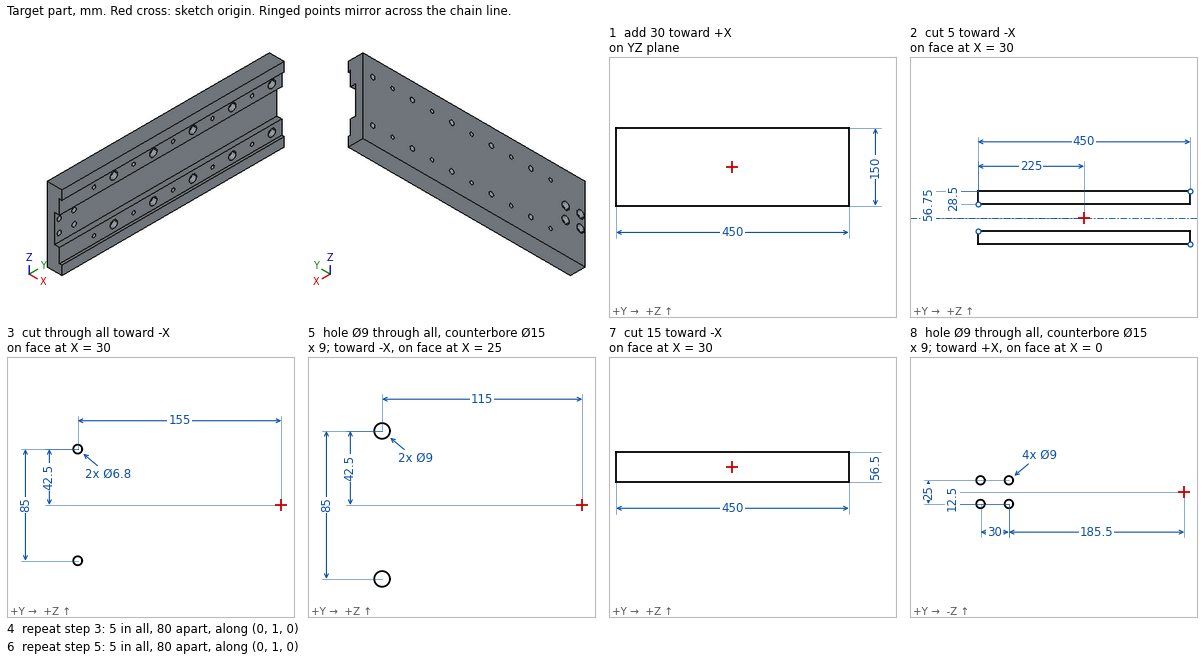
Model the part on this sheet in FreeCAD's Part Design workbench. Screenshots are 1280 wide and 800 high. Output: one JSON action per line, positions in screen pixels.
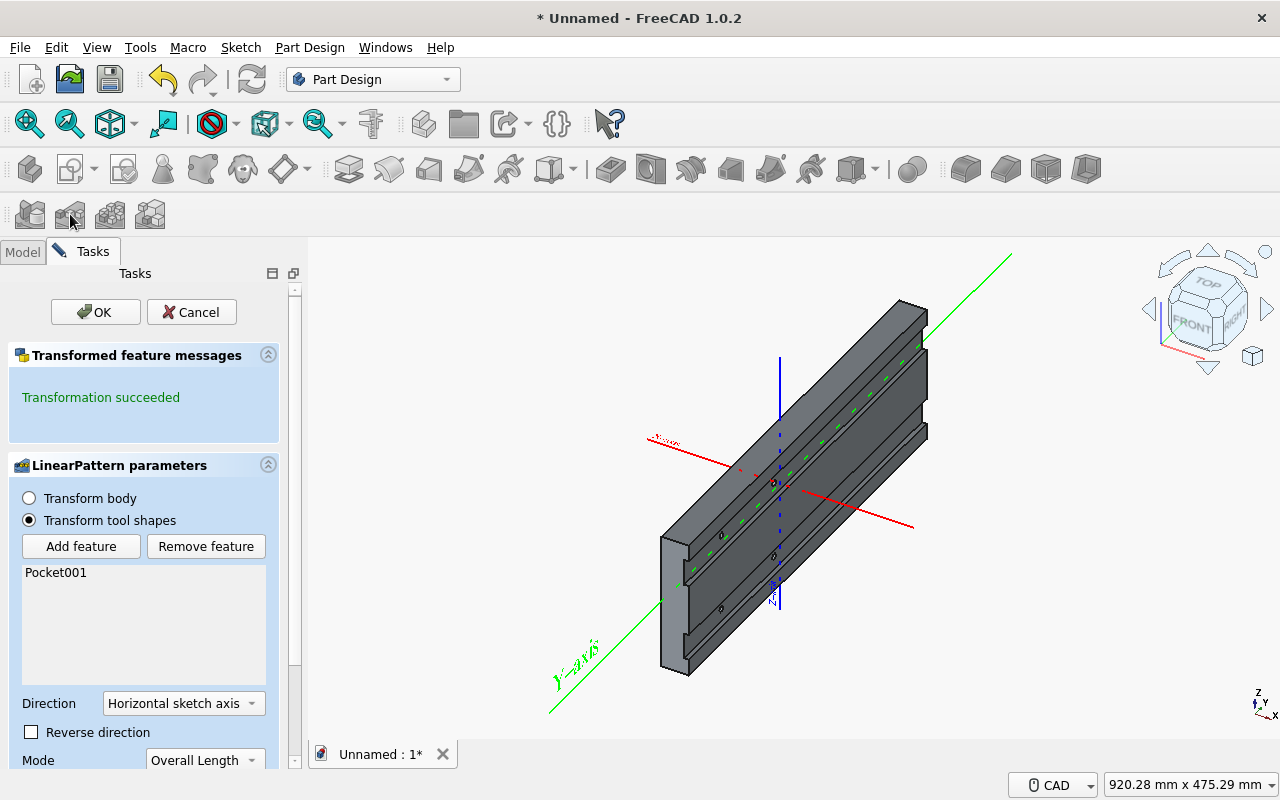
{"action": "left_click", "coordinate": [184, 704]}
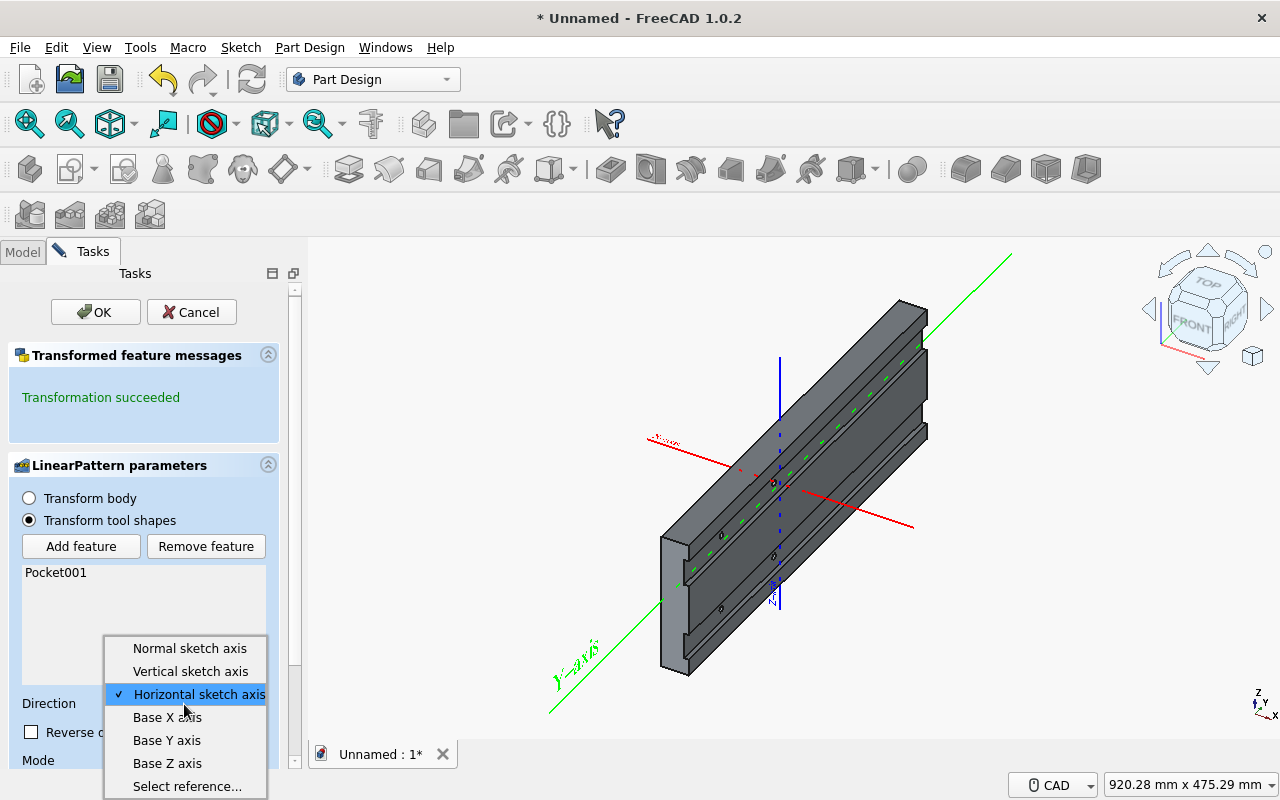
{"action": "left_click", "coordinate": [184, 740]}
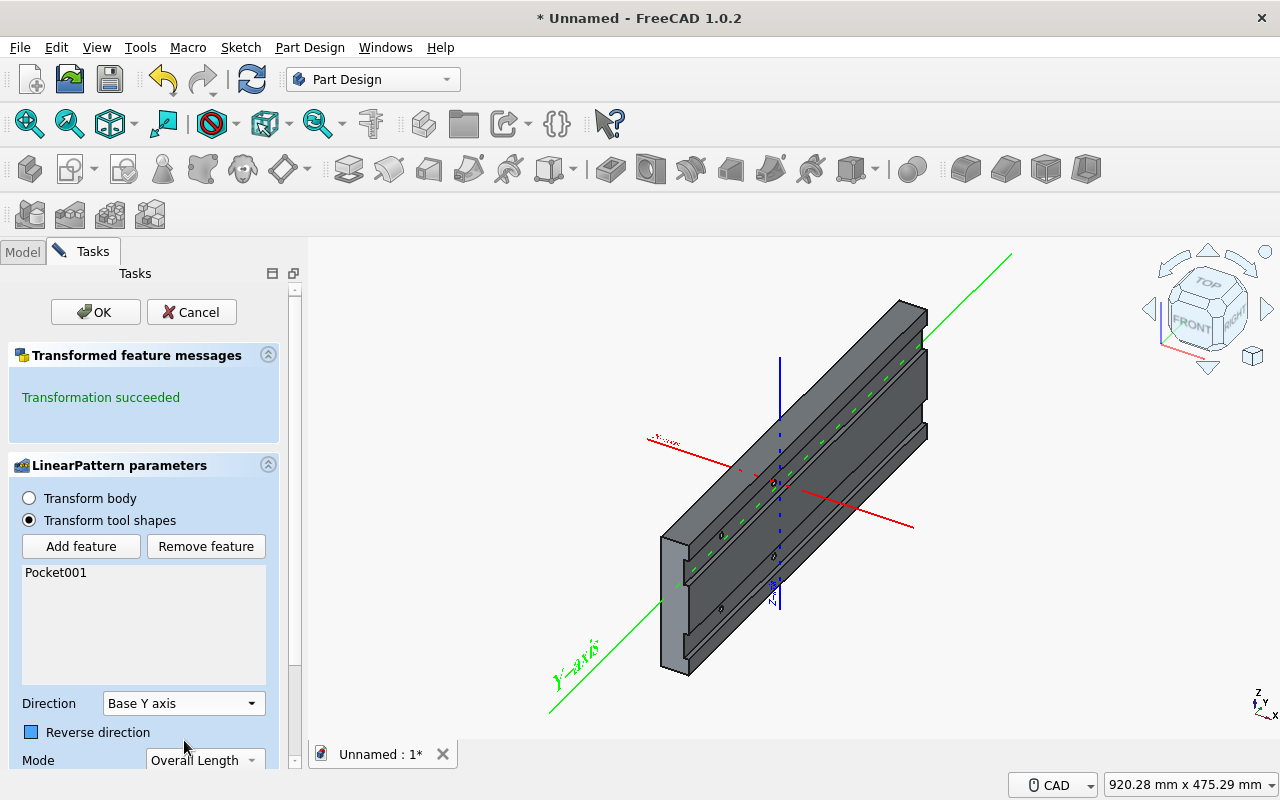
{"action": "scroll", "coordinate": [295, 526], "scroll_direction": "down", "scroll_amount": 2}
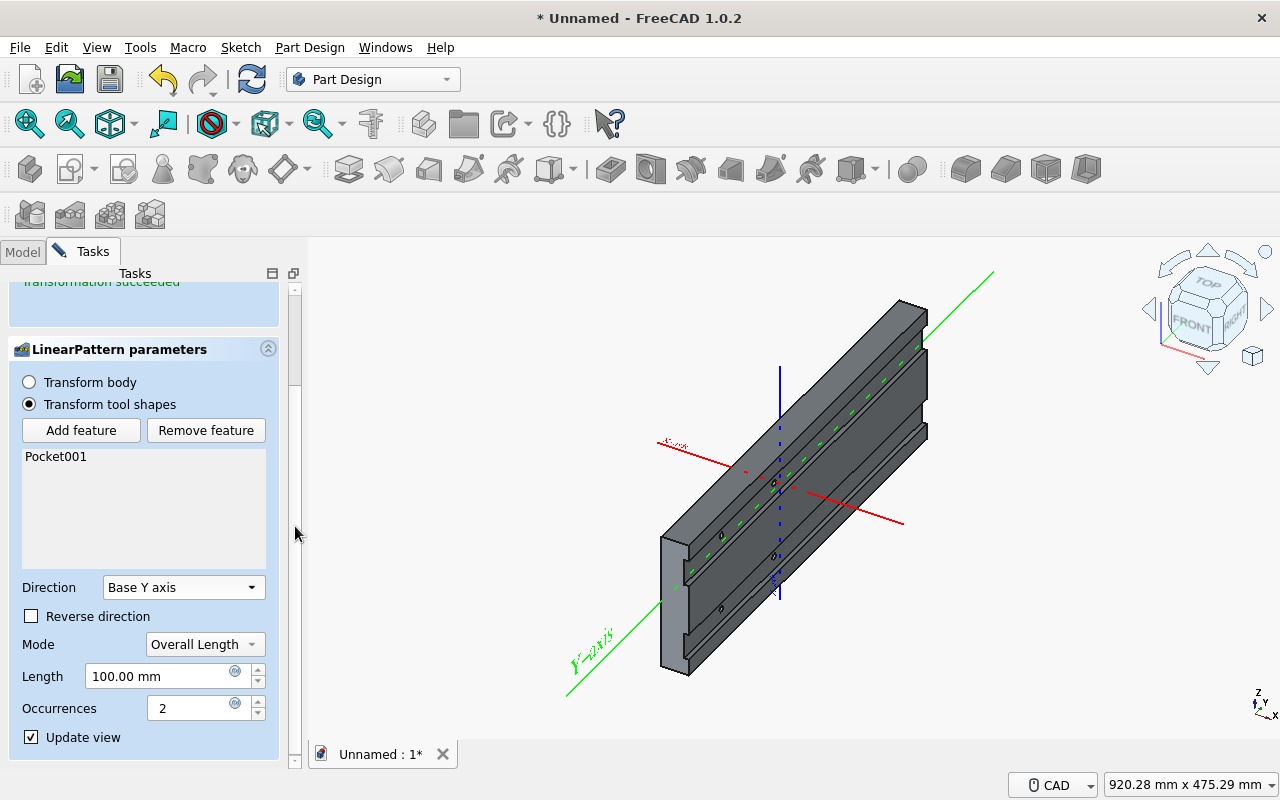
{"action": "left_click", "coordinate": [206, 644]}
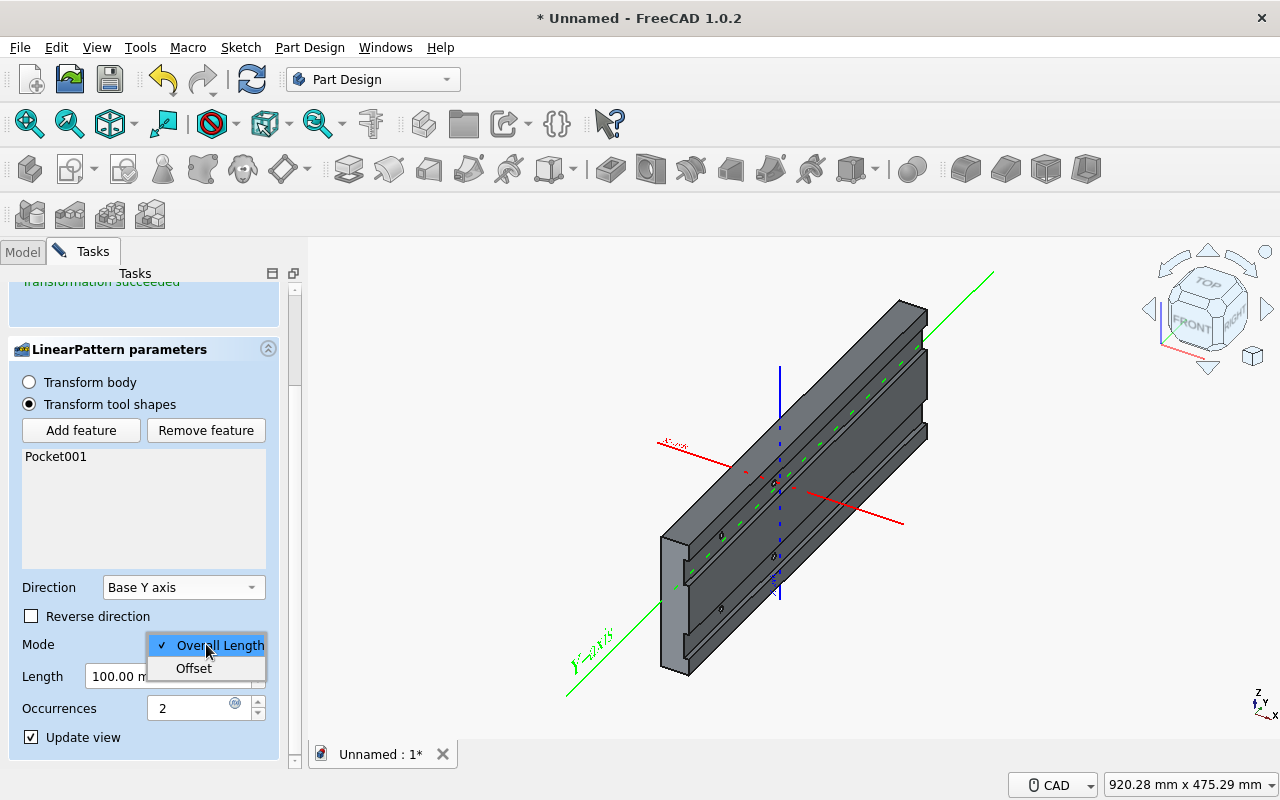
{"action": "left_click", "coordinate": [206, 668]}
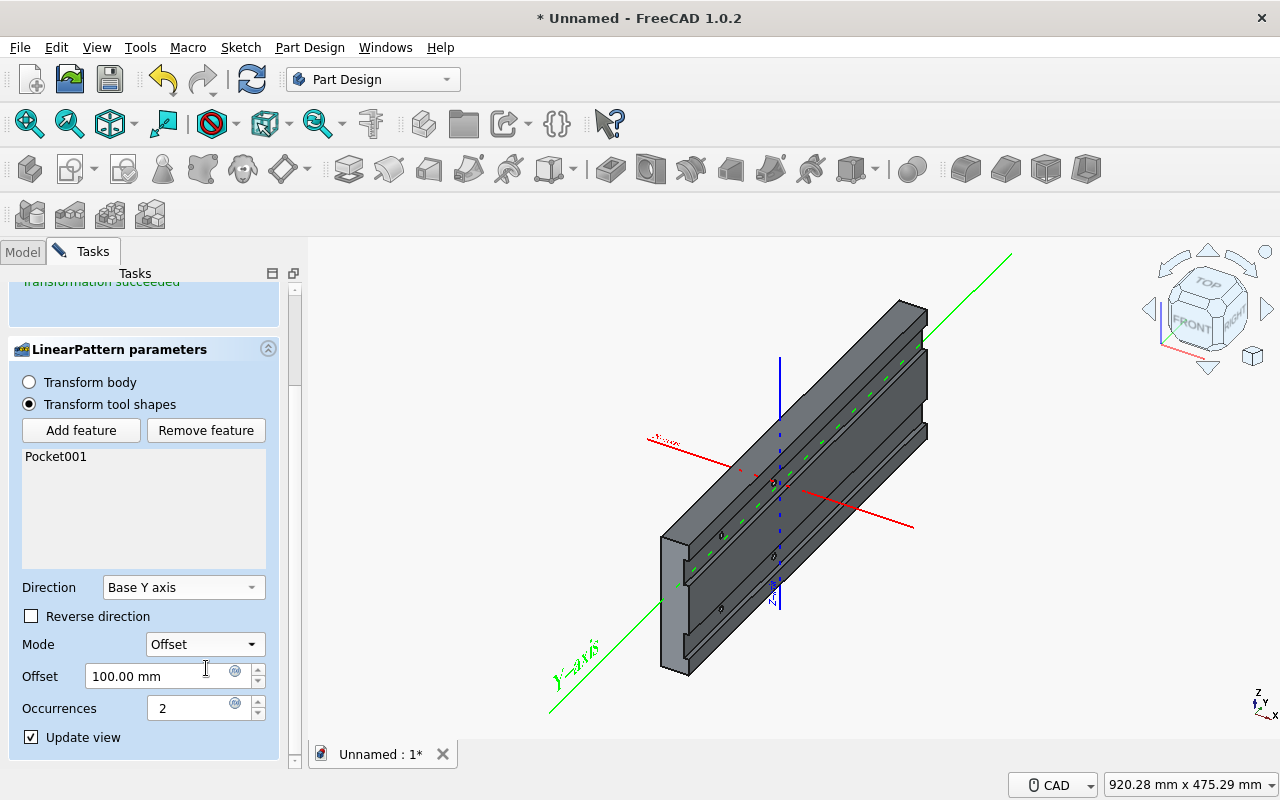
{"action": "triple_click", "coordinate": [168, 676]}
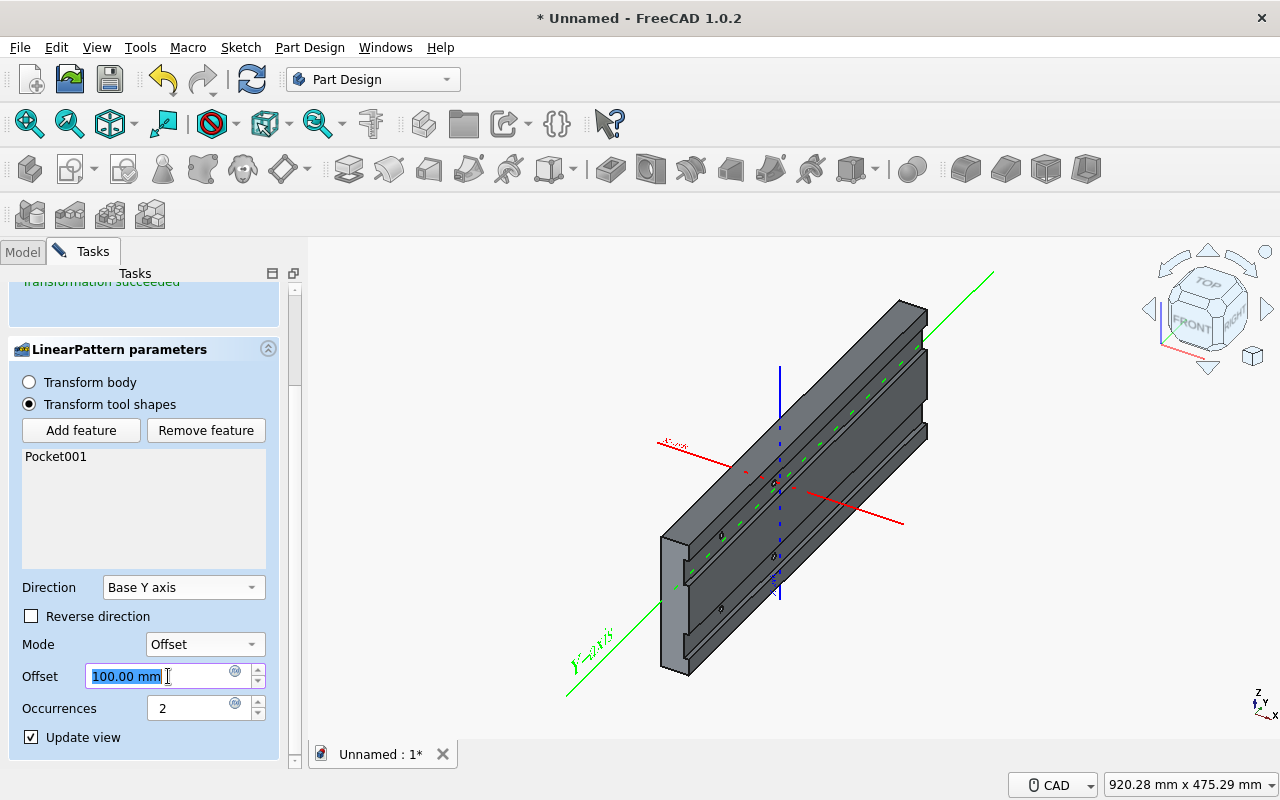
{"action": "type", "text": "80"}
{"action": "key", "text": "Tab"}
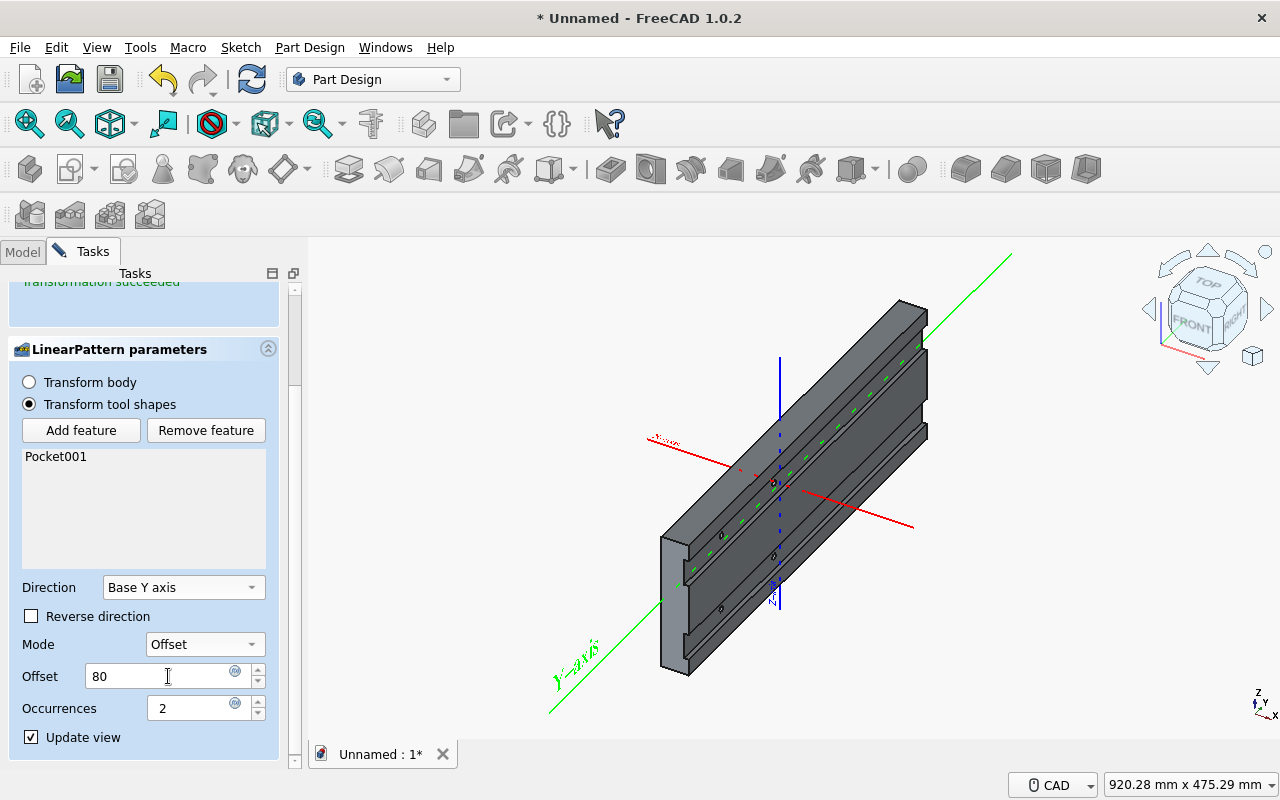
{"action": "triple_click", "coordinate": [198, 708]}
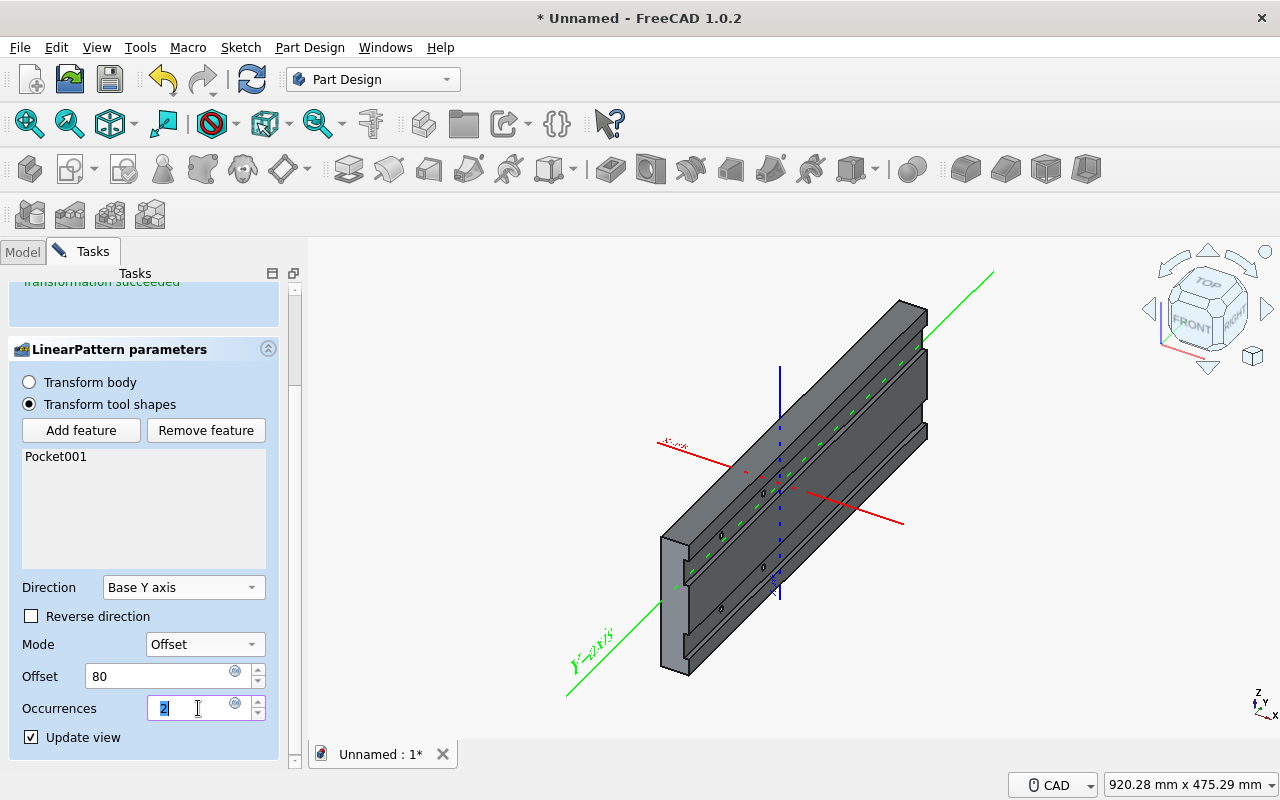
{"action": "type", "text": "5"}
{"action": "key", "text": "Tab"}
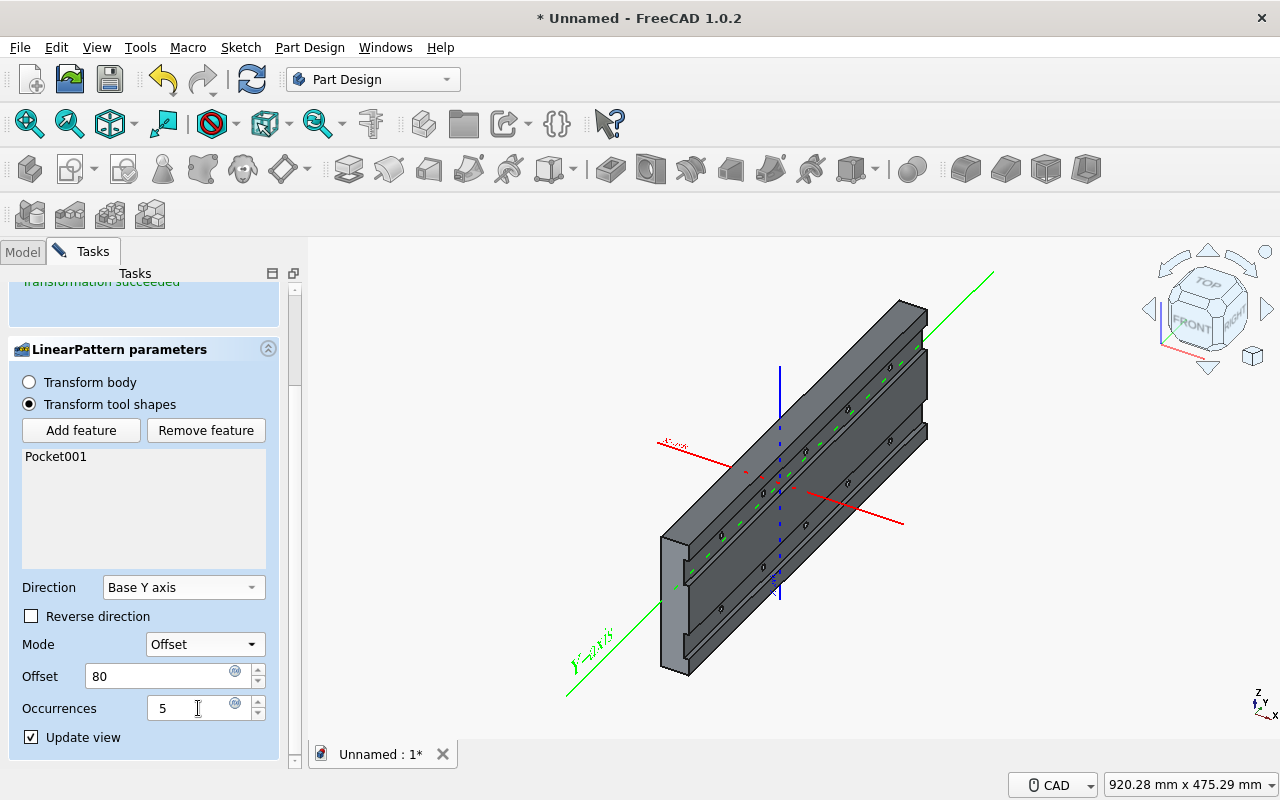
{"action": "scroll", "coordinate": [295, 526], "scroll_direction": "up", "scroll_amount": 3}